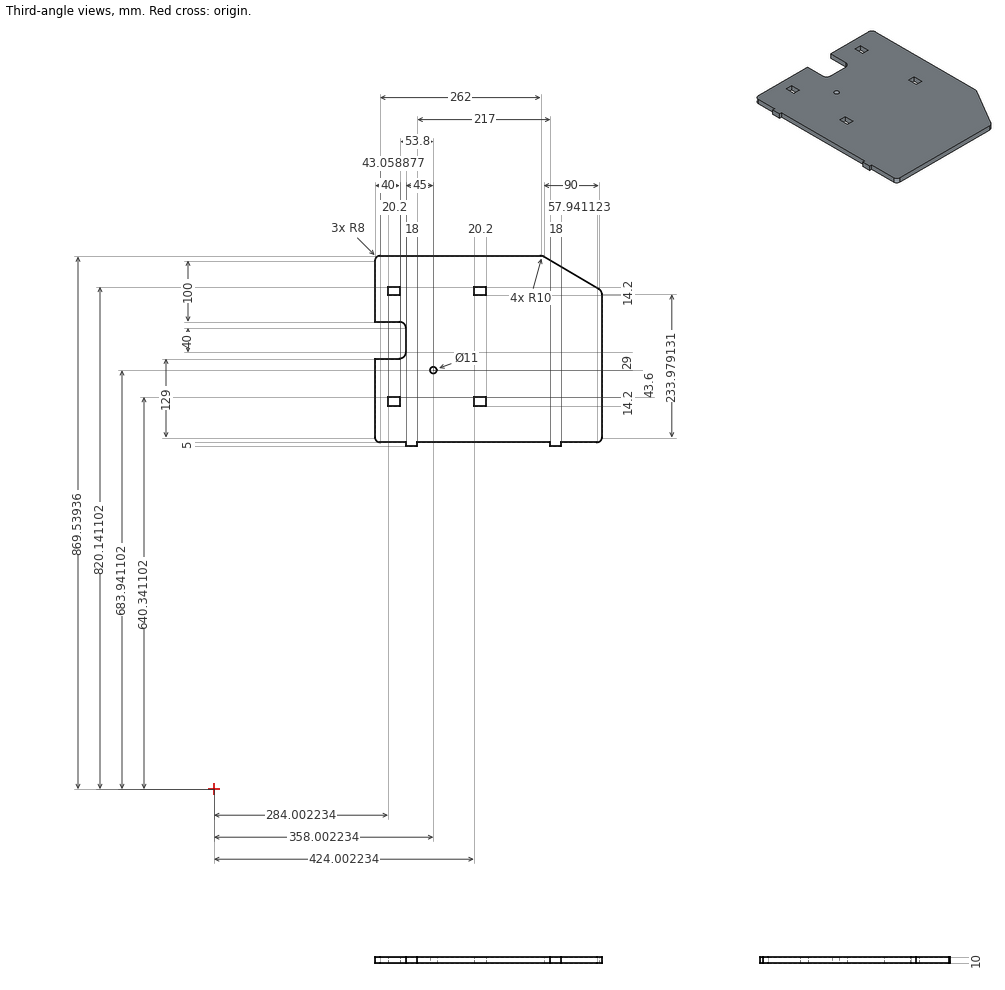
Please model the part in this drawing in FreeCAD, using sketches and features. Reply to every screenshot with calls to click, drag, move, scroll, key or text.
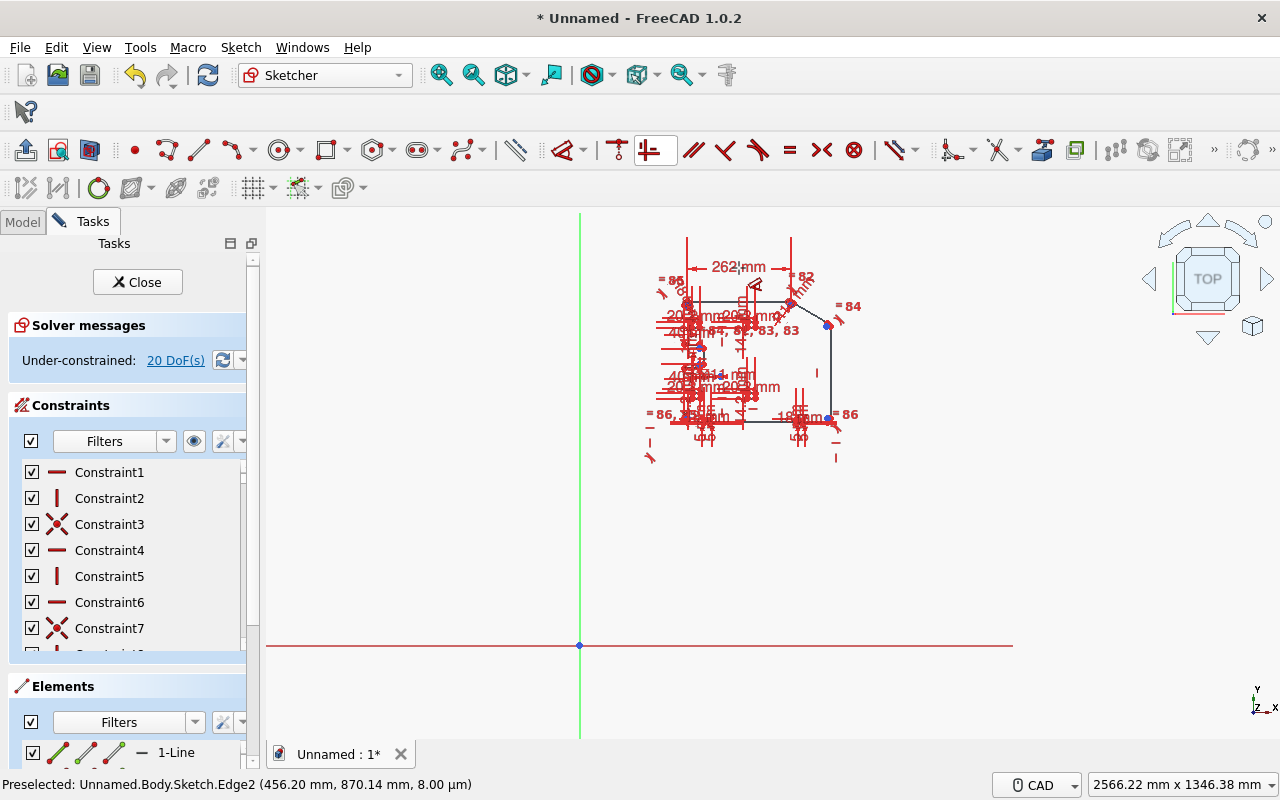
scroll(684, 317, up, 3)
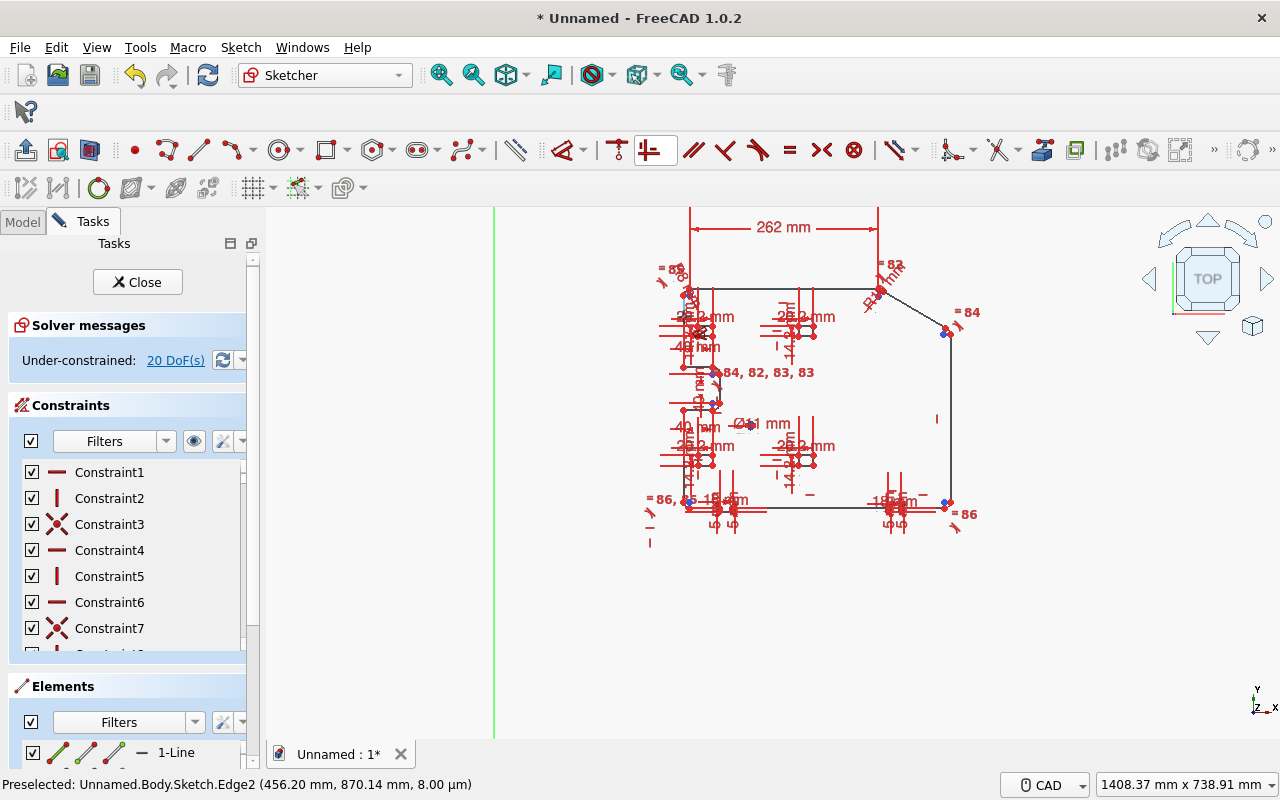
click(684, 317)
click(650, 315)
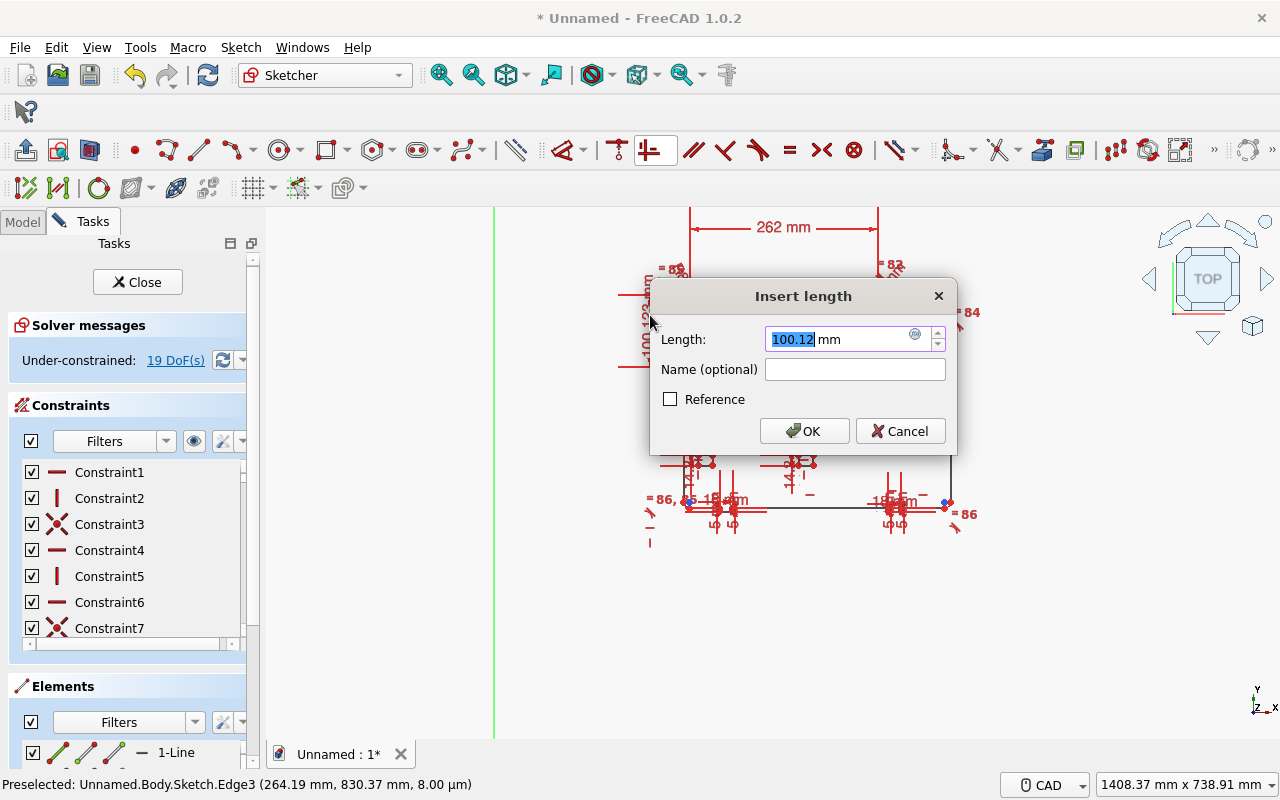
text(100)
key(Return)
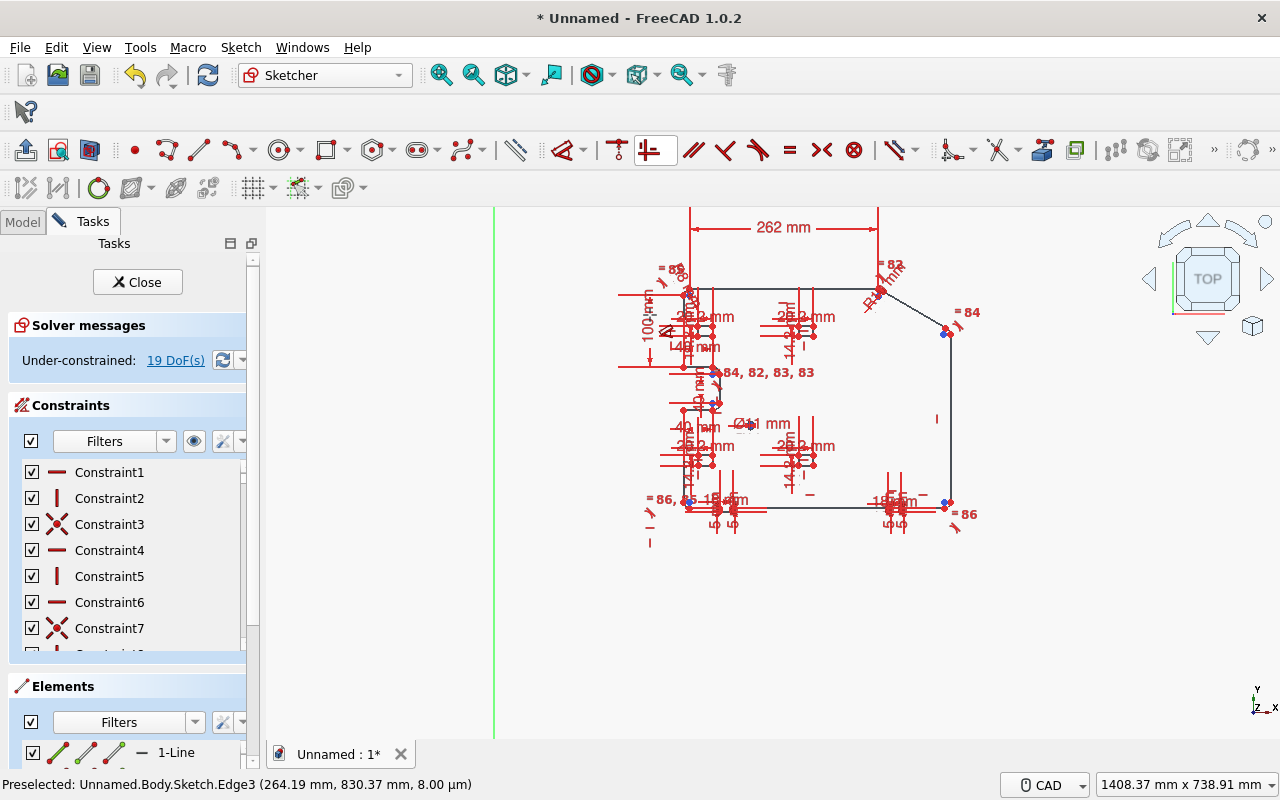
click(684, 438)
click(650, 456)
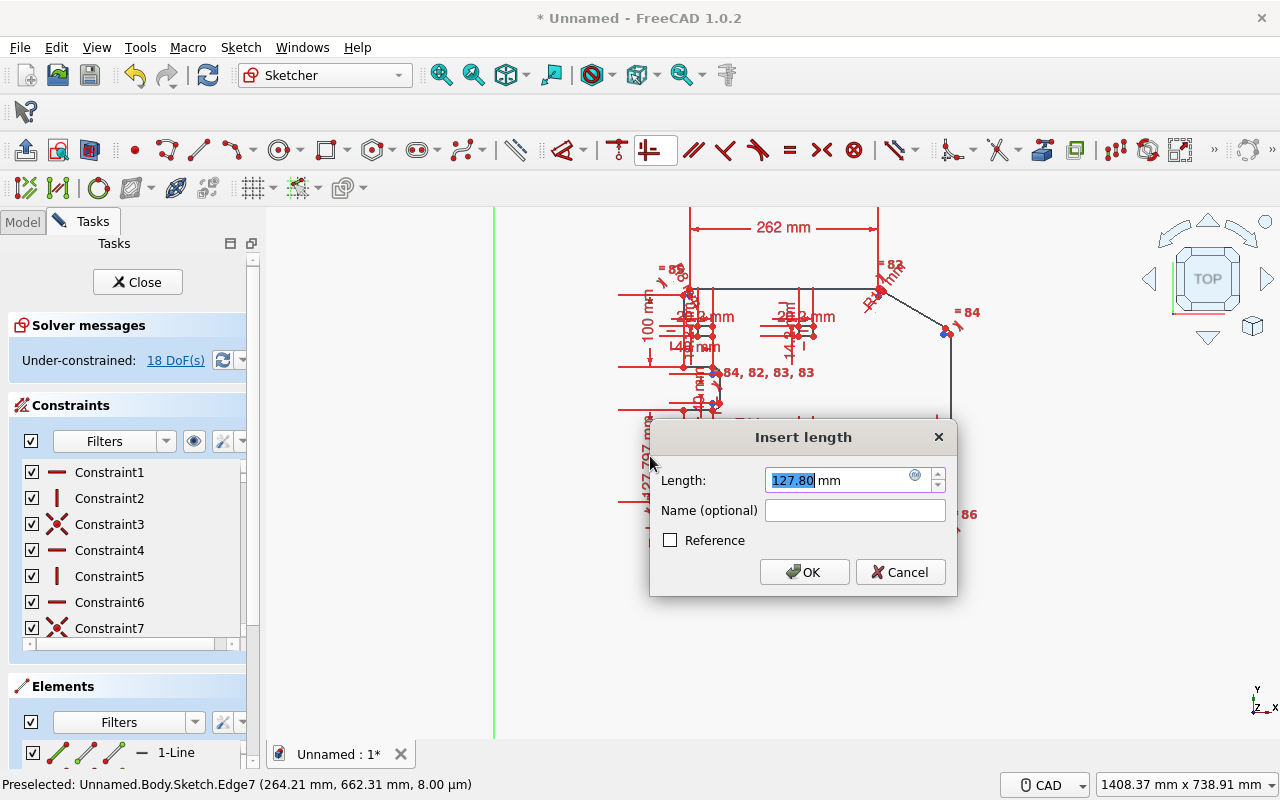
text(129)
key(Return)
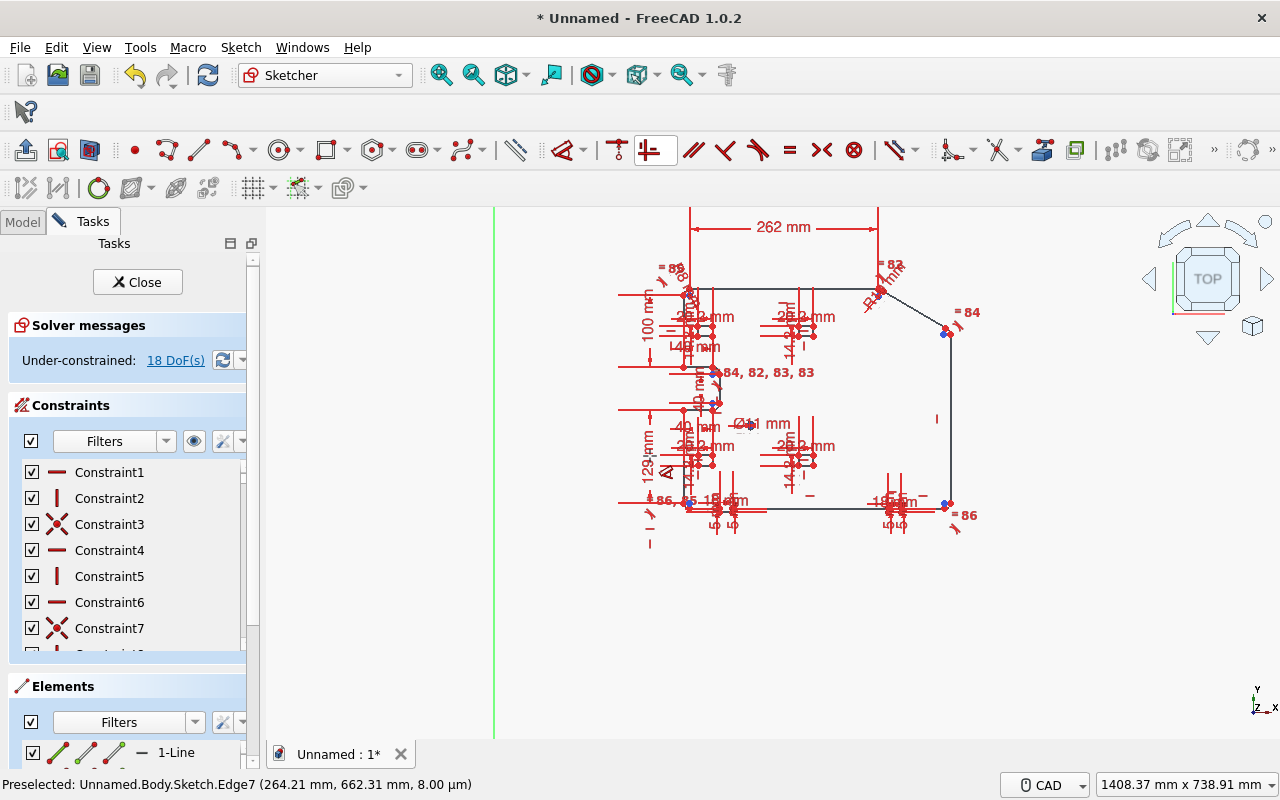
click(779, 509)
click(775, 475)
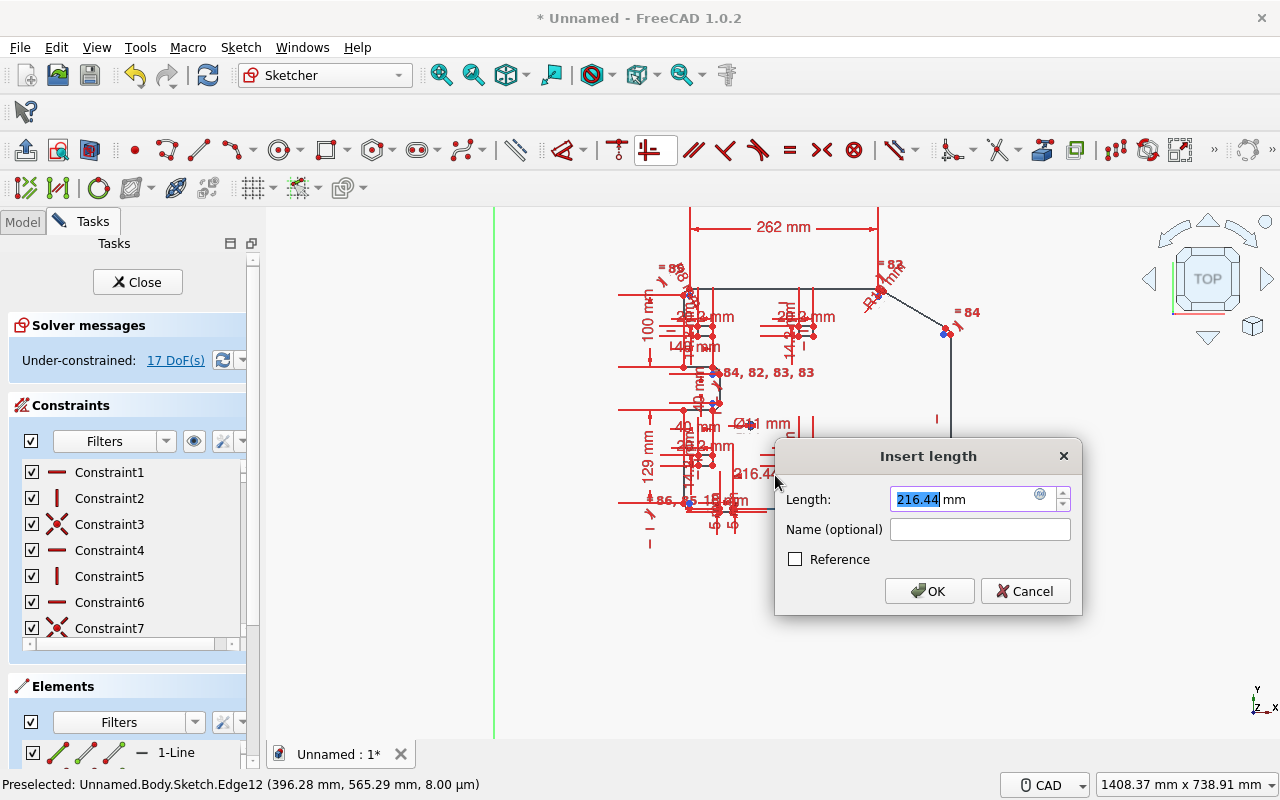
text(217)
key(Return)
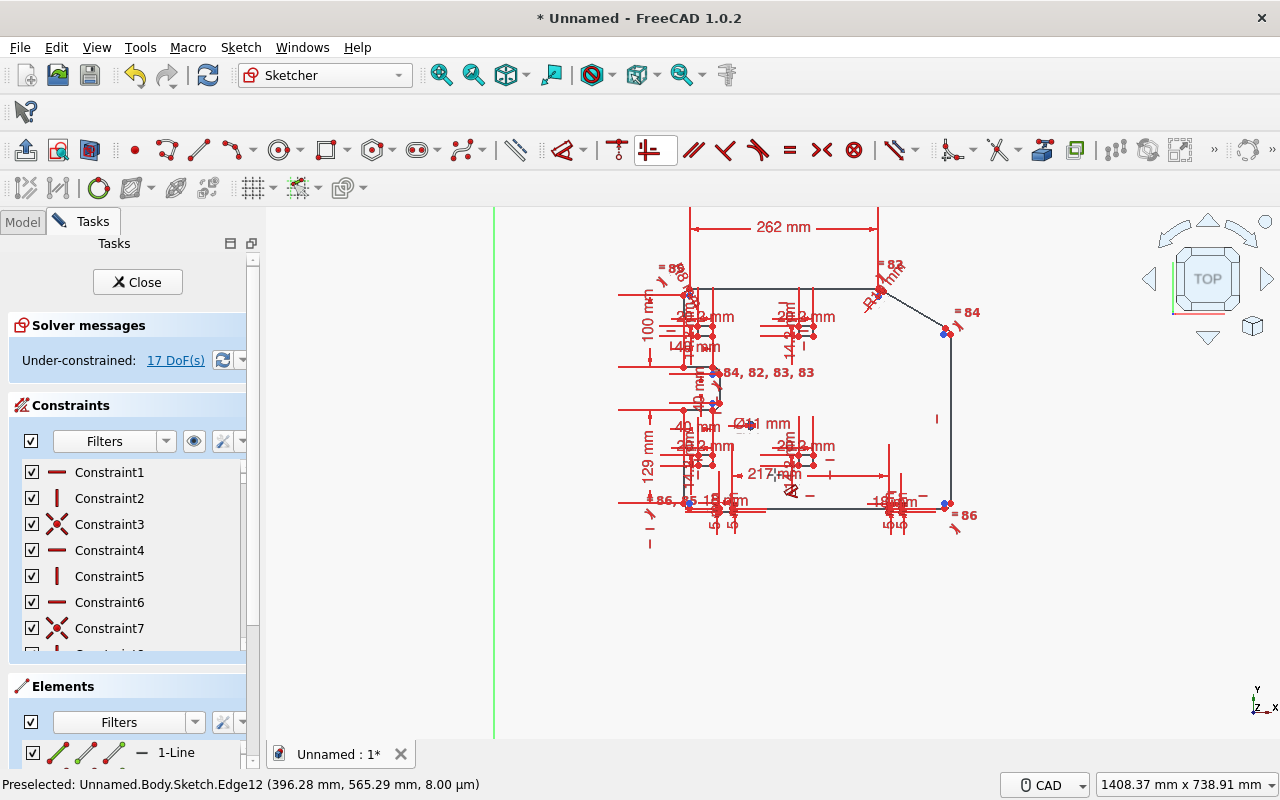
click(927, 317)
click(915, 257)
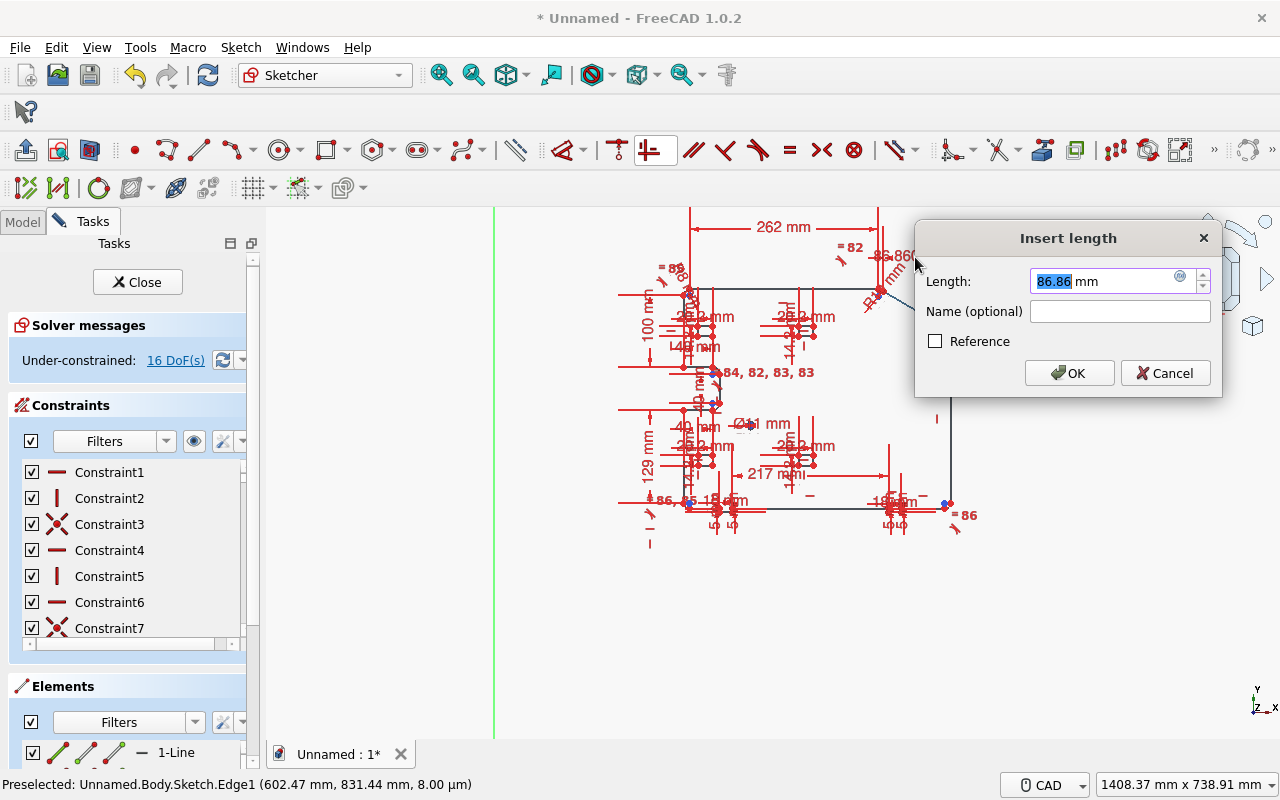
text(90)
key(Return)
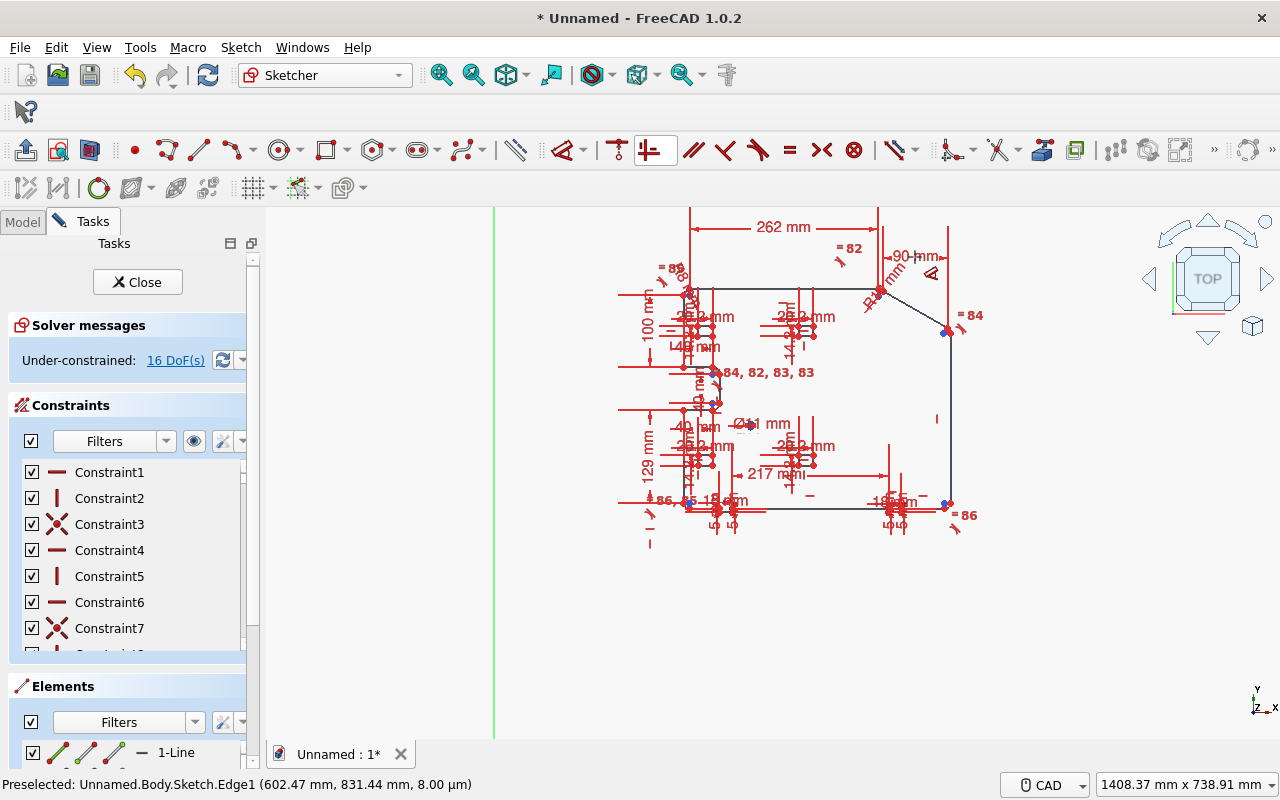
scroll(720, 403, up, 3)